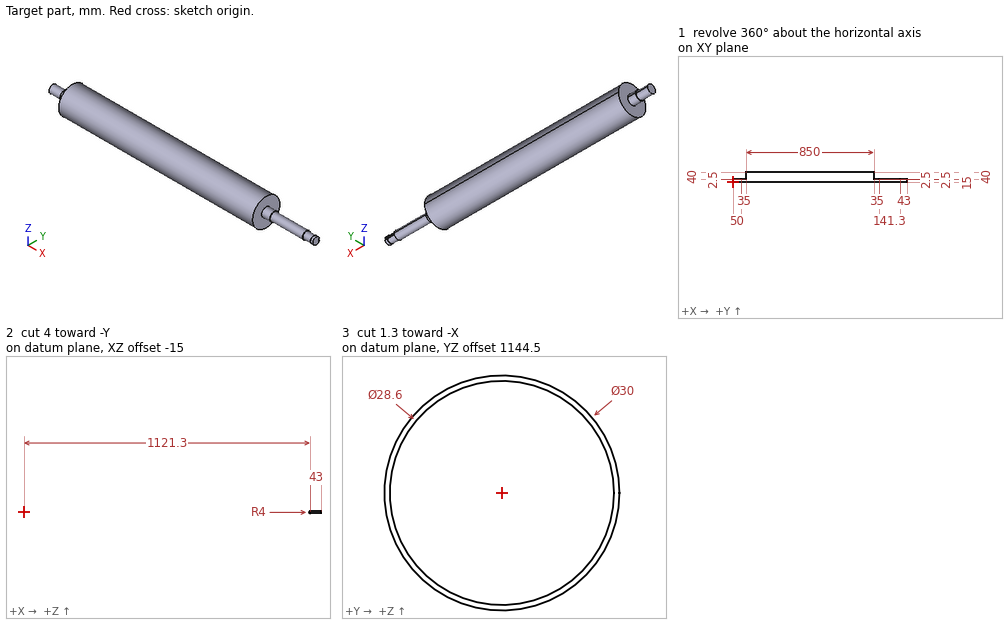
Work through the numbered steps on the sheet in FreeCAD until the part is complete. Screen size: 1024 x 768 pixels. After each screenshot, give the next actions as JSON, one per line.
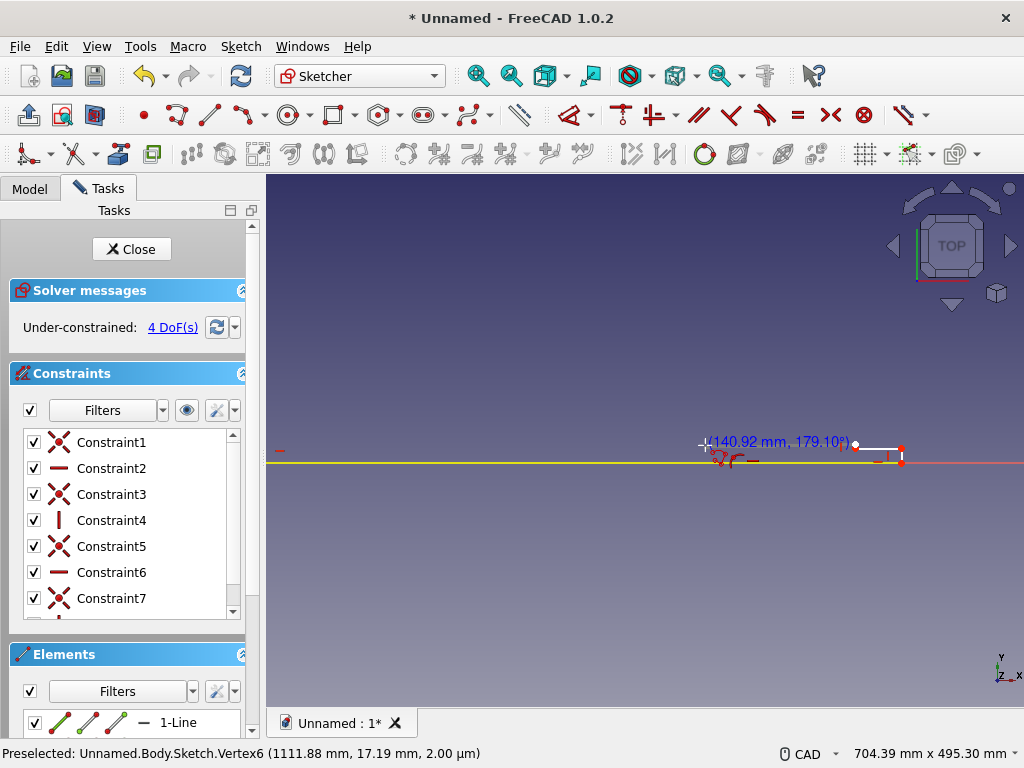
{"action": "left_click", "coordinate": [703, 445]}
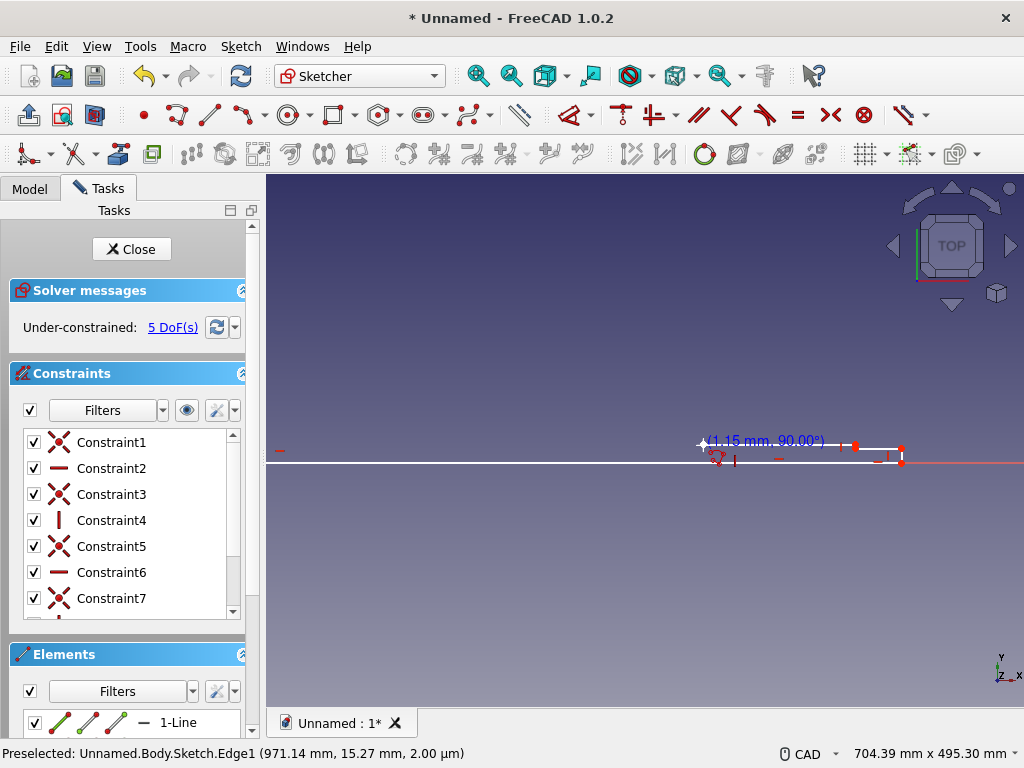
{"action": "scroll", "coordinate": [703, 442], "scroll_direction": "up", "scroll_amount": 9}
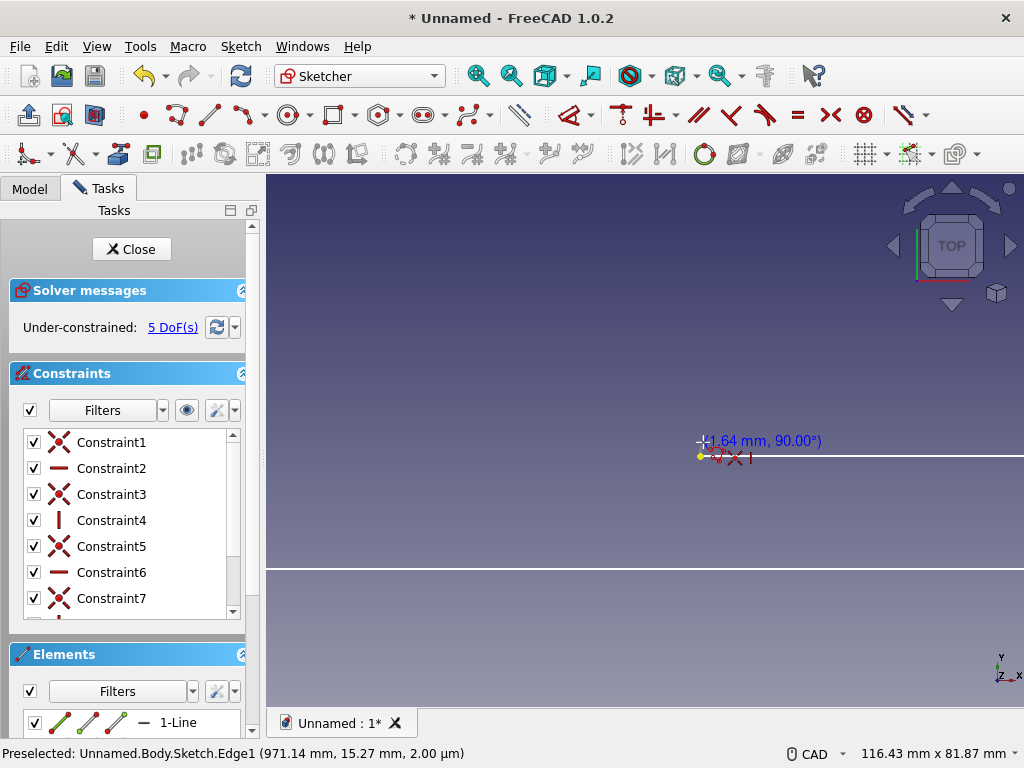
{"action": "left_click", "coordinate": [700, 439]}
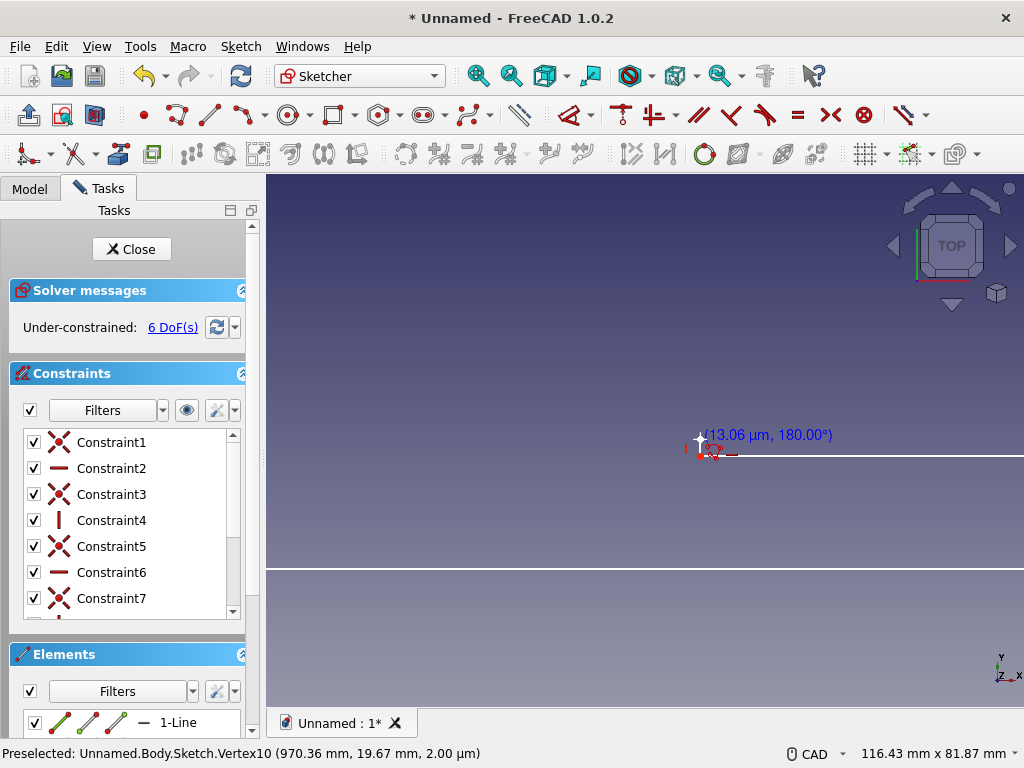
{"action": "scroll", "coordinate": [704, 444], "scroll_direction": "down", "scroll_amount": 15}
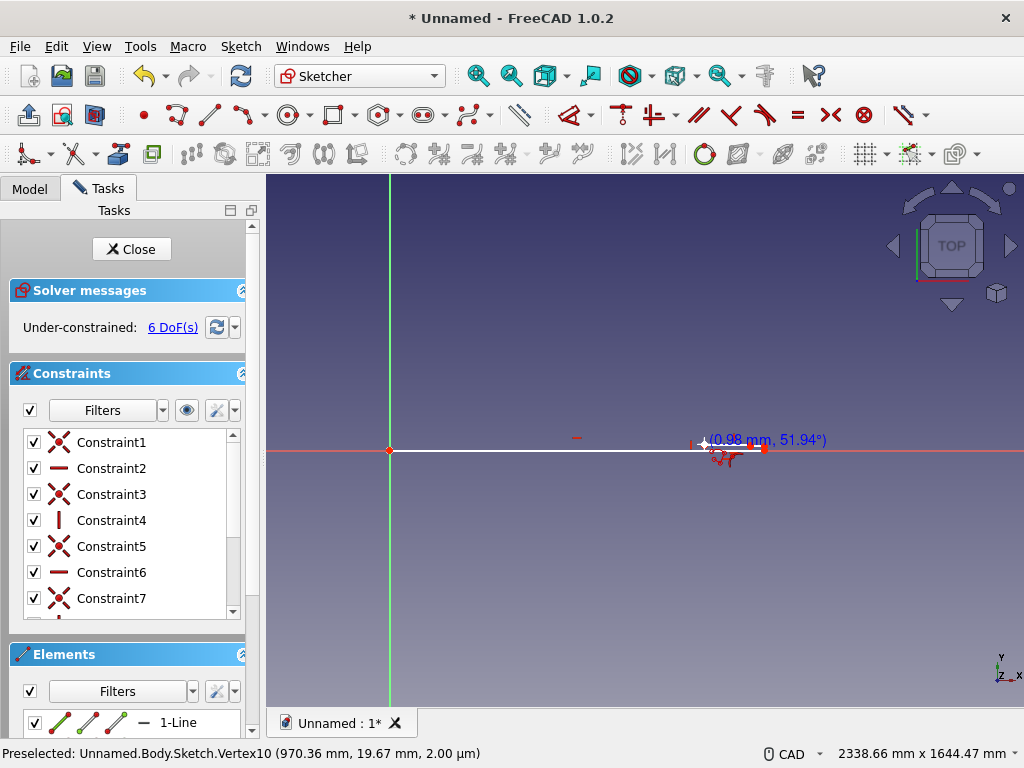
{"action": "scroll", "coordinate": [693, 444], "scroll_direction": "up", "scroll_amount": 5}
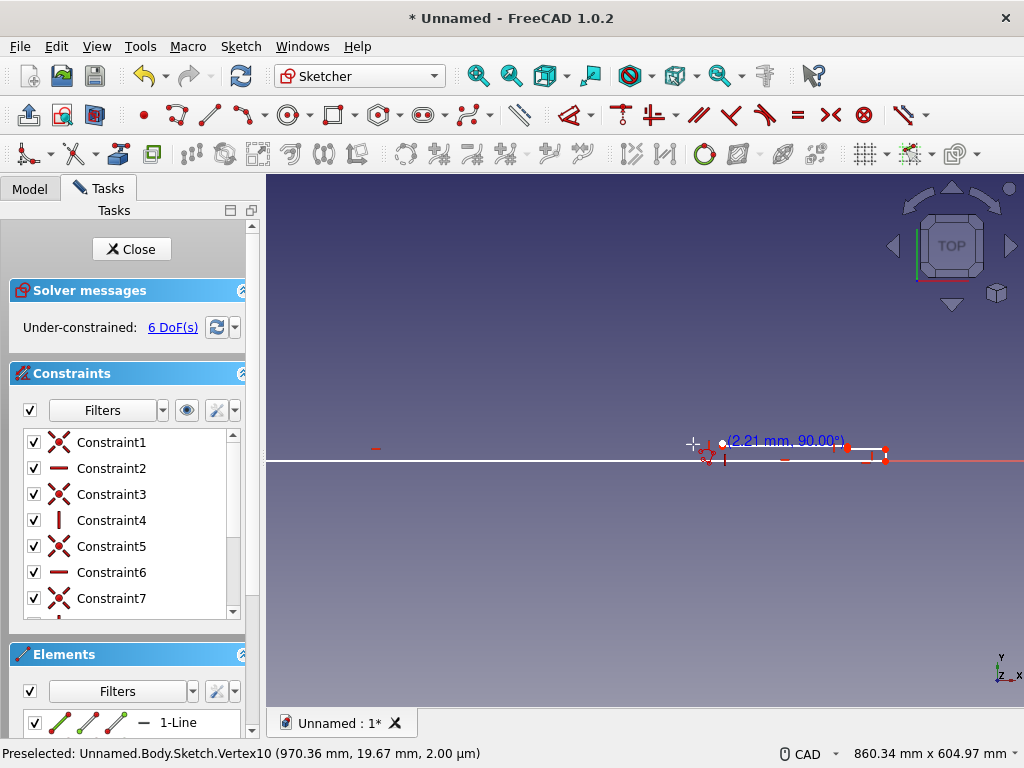
{"action": "left_click", "coordinate": [692, 444]}
{"action": "left_click", "coordinate": [692, 409]}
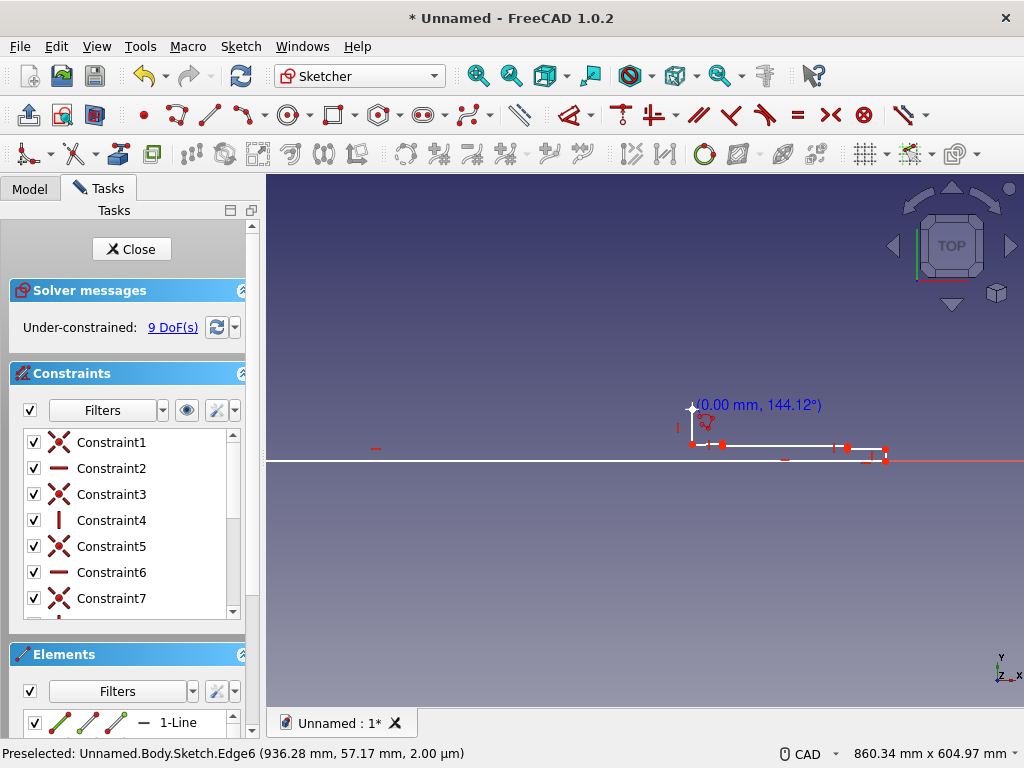
{"action": "scroll", "coordinate": [693, 444], "scroll_direction": "down", "scroll_amount": 5}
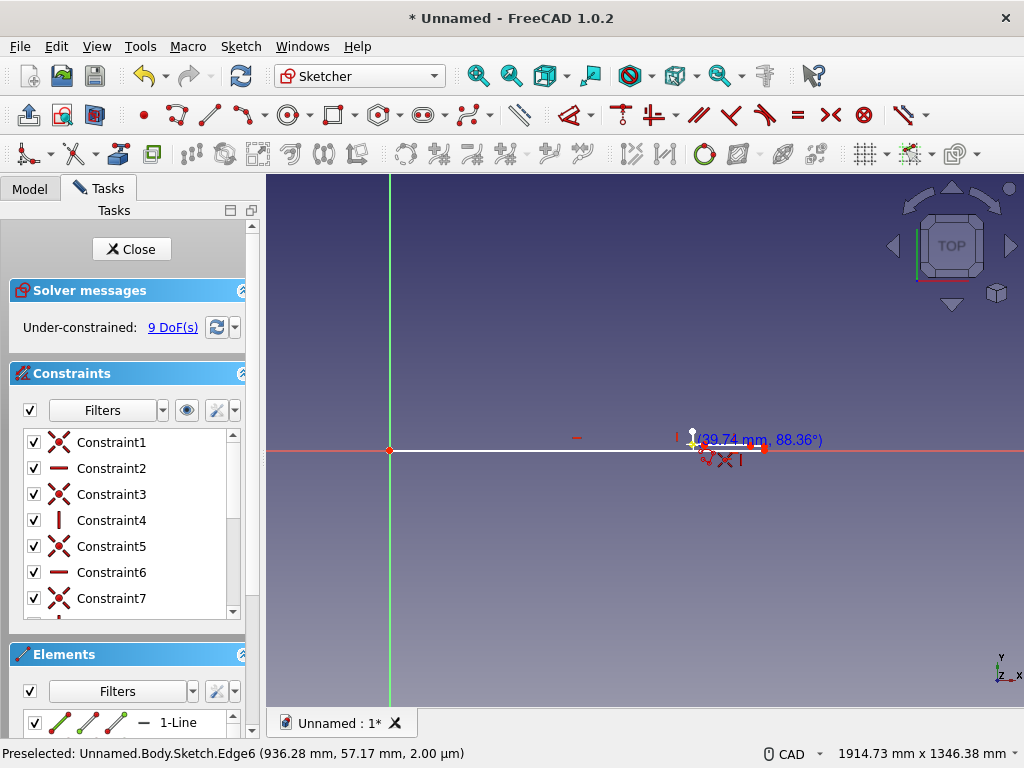
{"action": "left_click", "coordinate": [417, 431]}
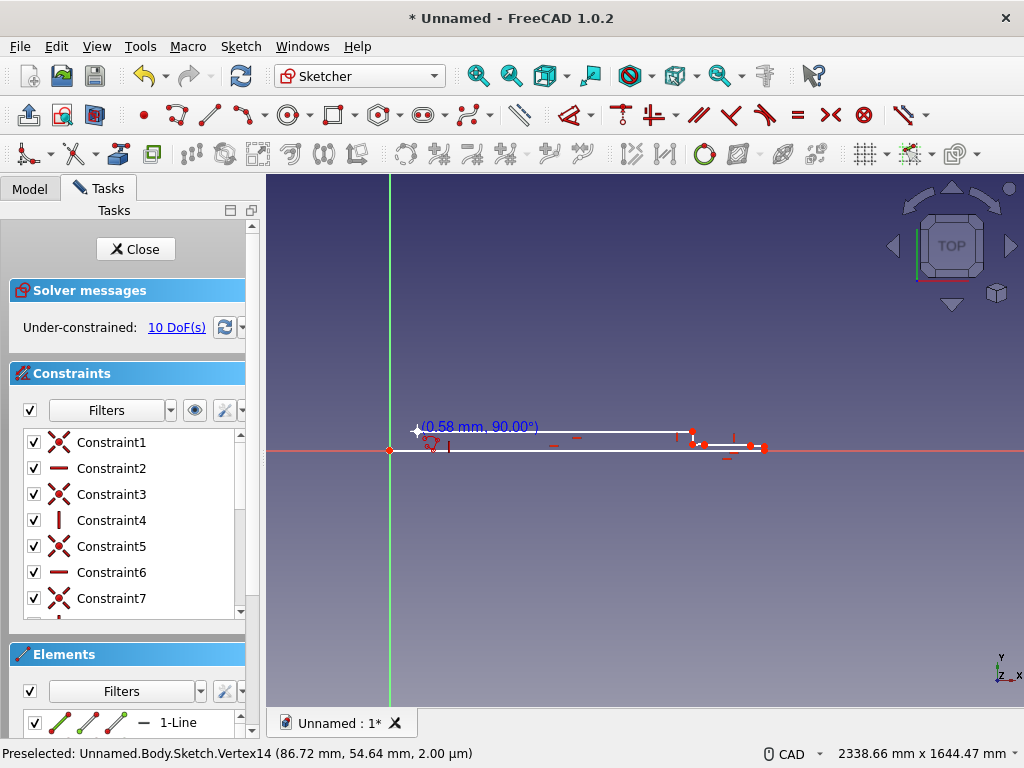
{"action": "scroll", "coordinate": [417, 444], "scroll_direction": "up", "scroll_amount": 5}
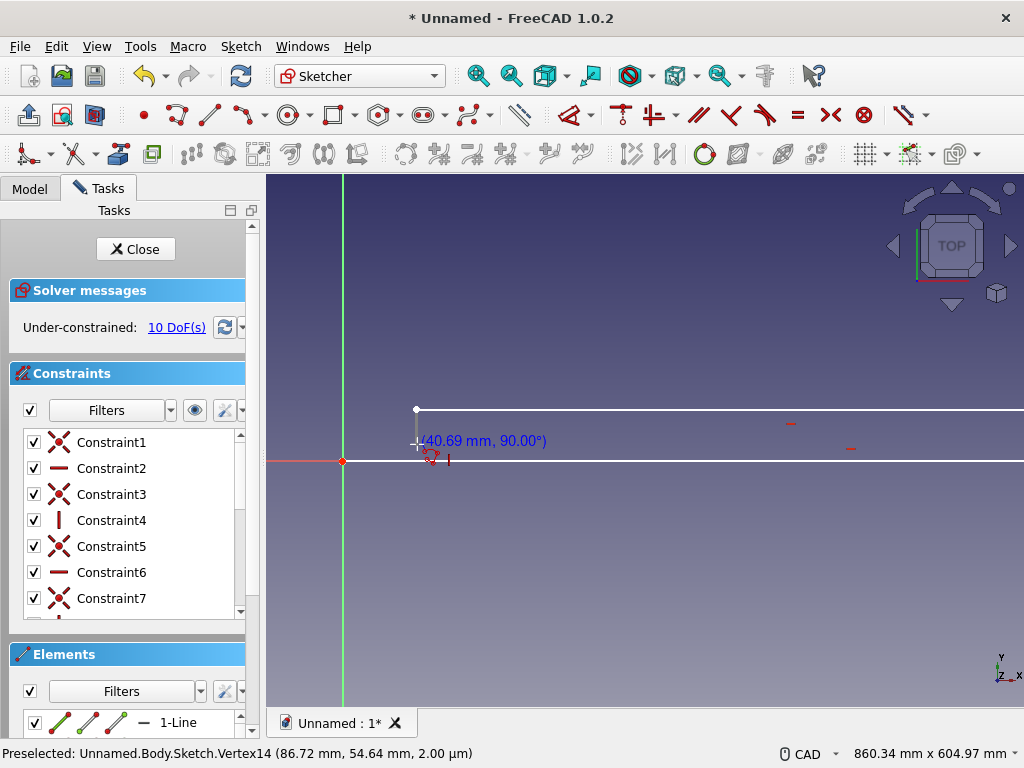
{"action": "left_click", "coordinate": [417, 444]}
{"action": "left_click", "coordinate": [387, 444]}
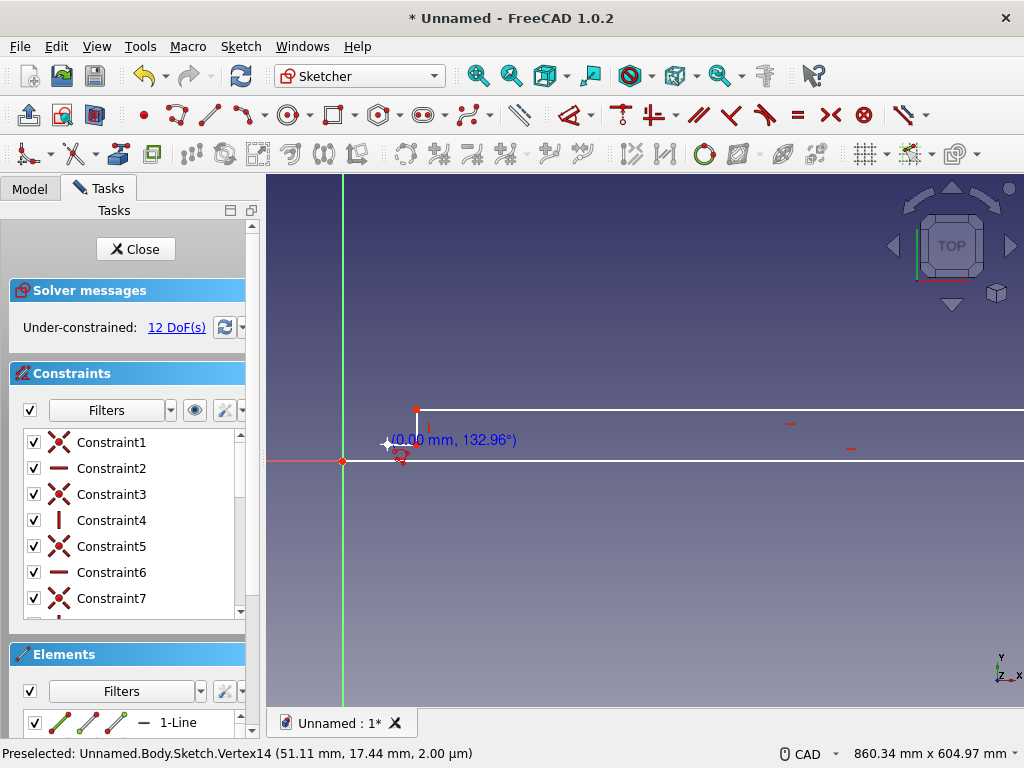
{"action": "scroll", "coordinate": [387, 446], "scroll_direction": "up", "scroll_amount": 10}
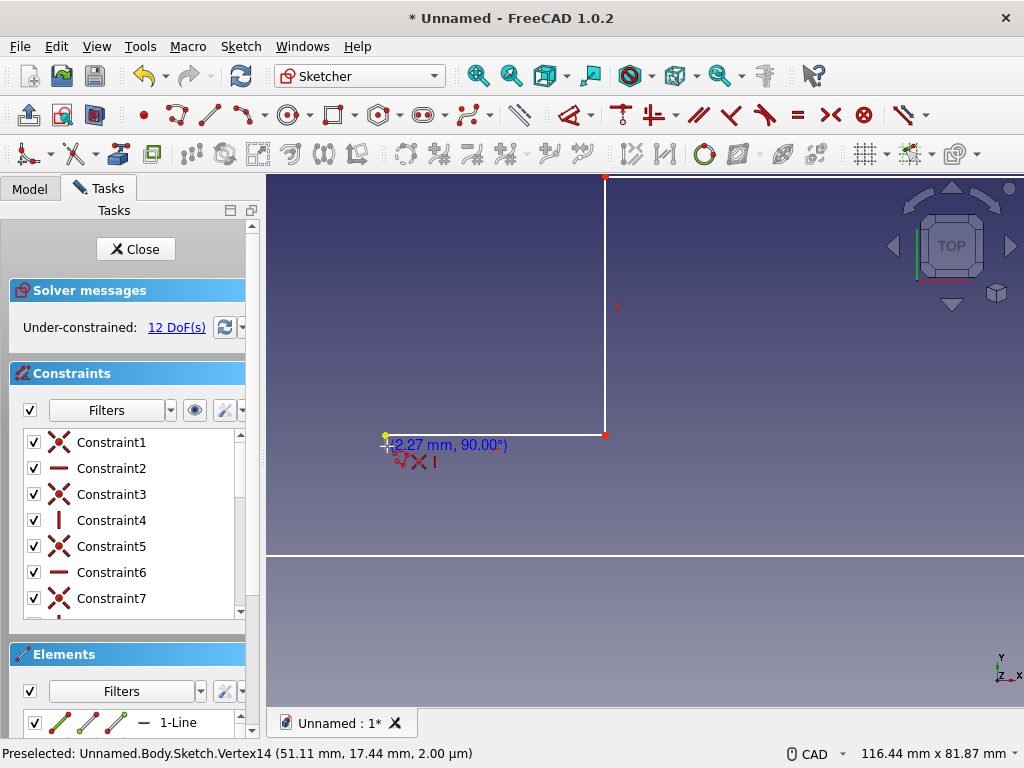
{"action": "left_click", "coordinate": [386, 442]}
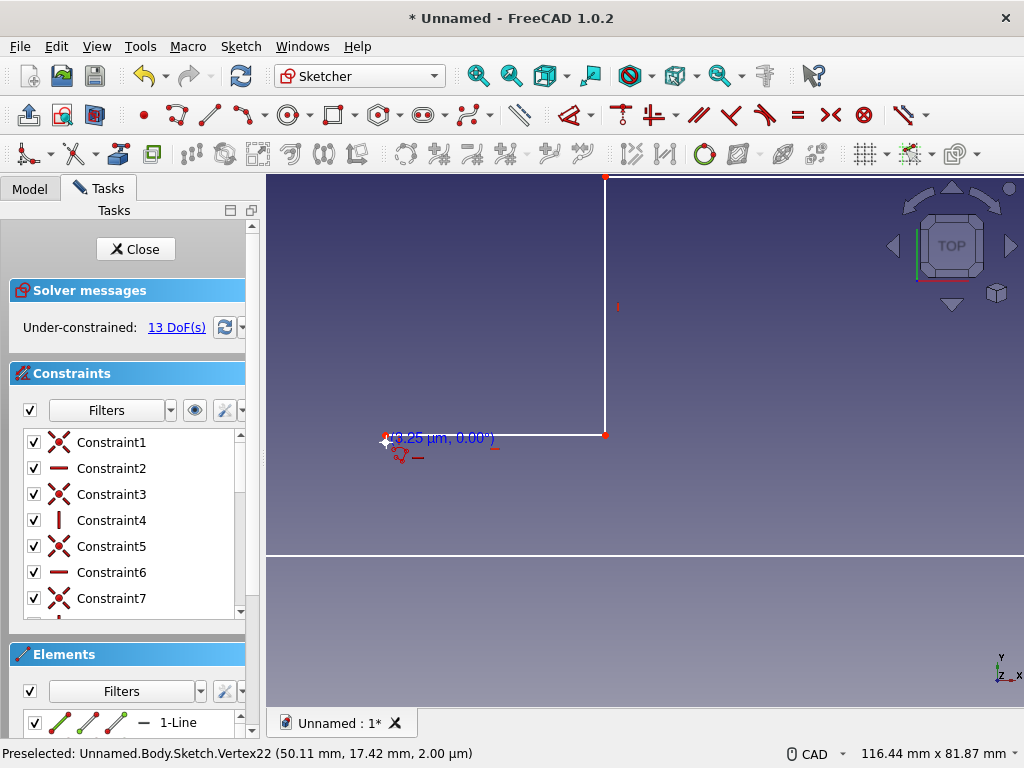
{"action": "scroll", "coordinate": [407, 445], "scroll_direction": "down", "scroll_amount": 15}